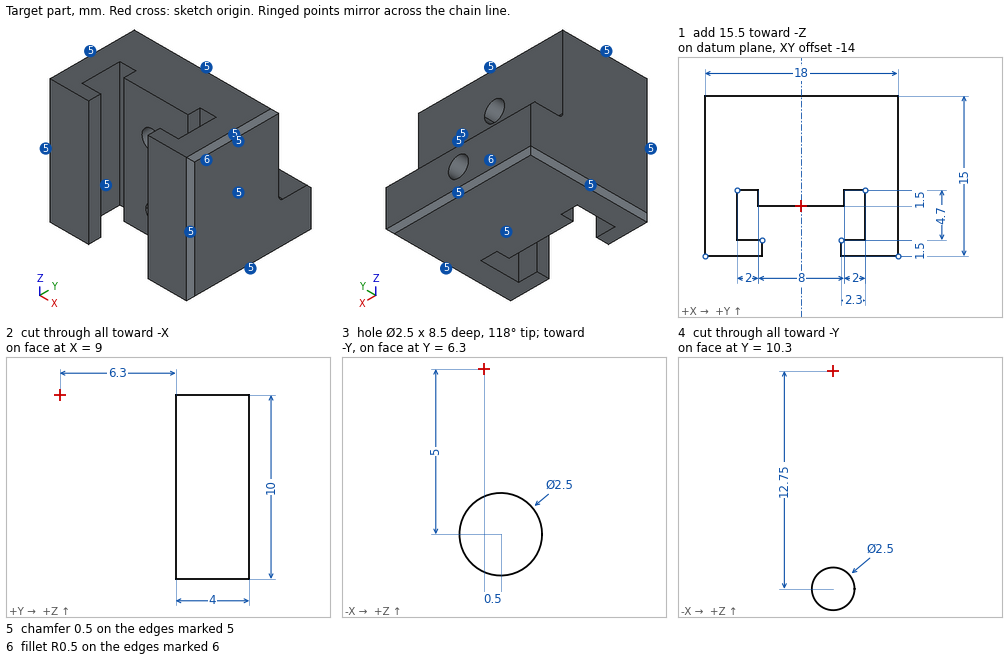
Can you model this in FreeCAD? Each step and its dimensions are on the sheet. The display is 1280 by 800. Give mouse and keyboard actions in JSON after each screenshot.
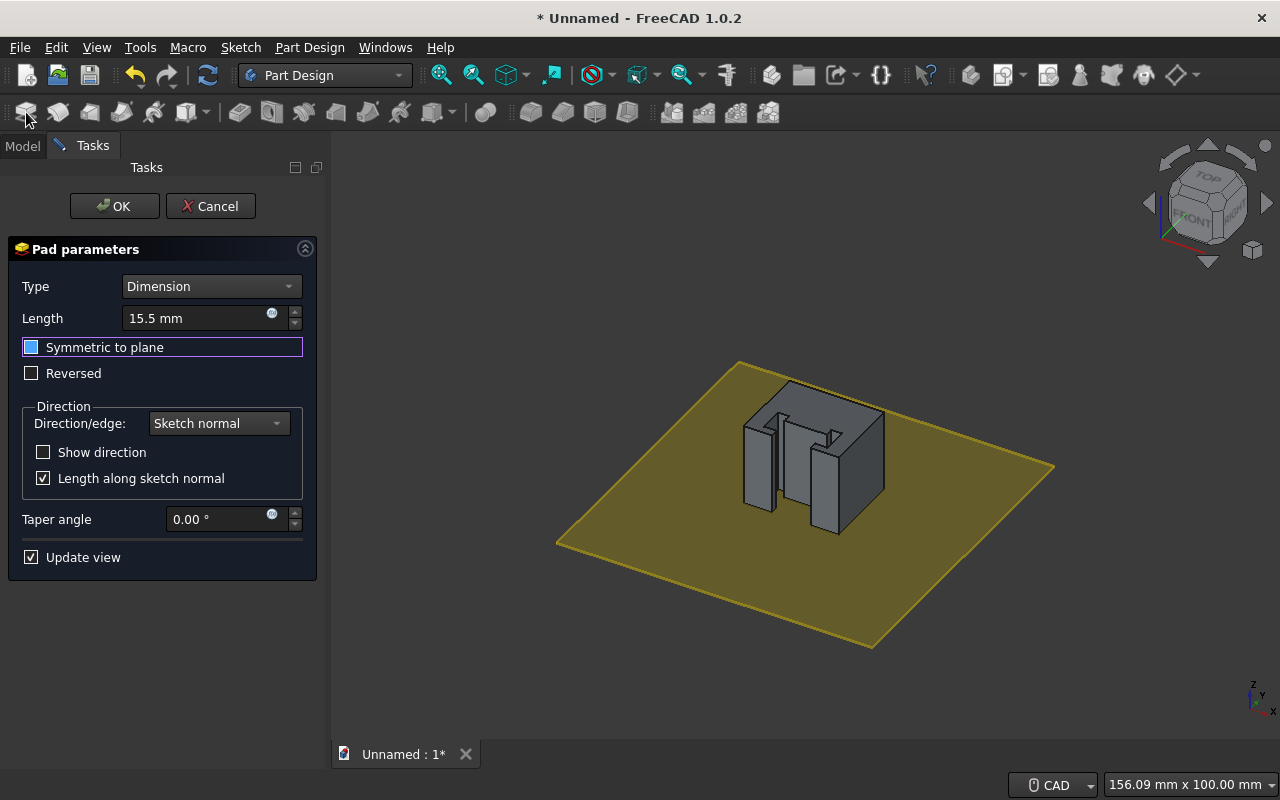
{"action": "left_click", "coordinate": [30, 373]}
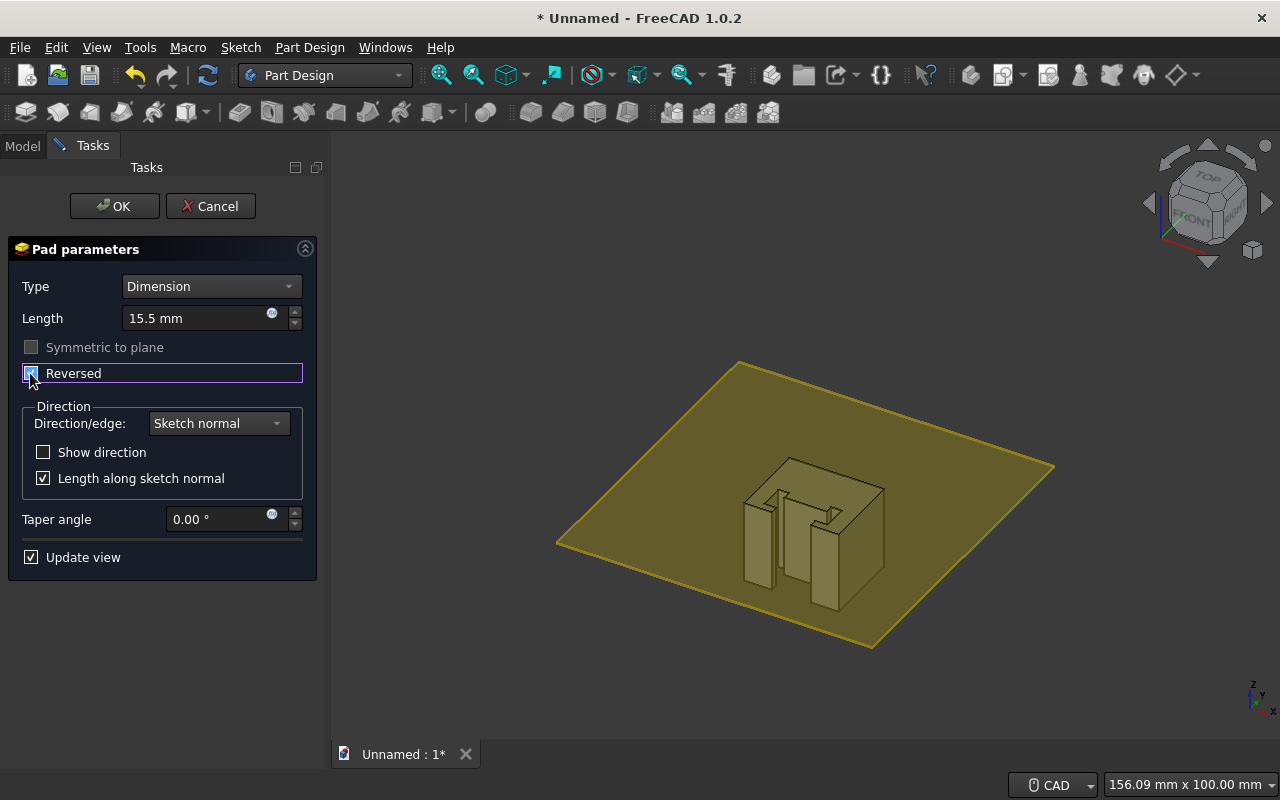
{"action": "left_click", "coordinate": [115, 206]}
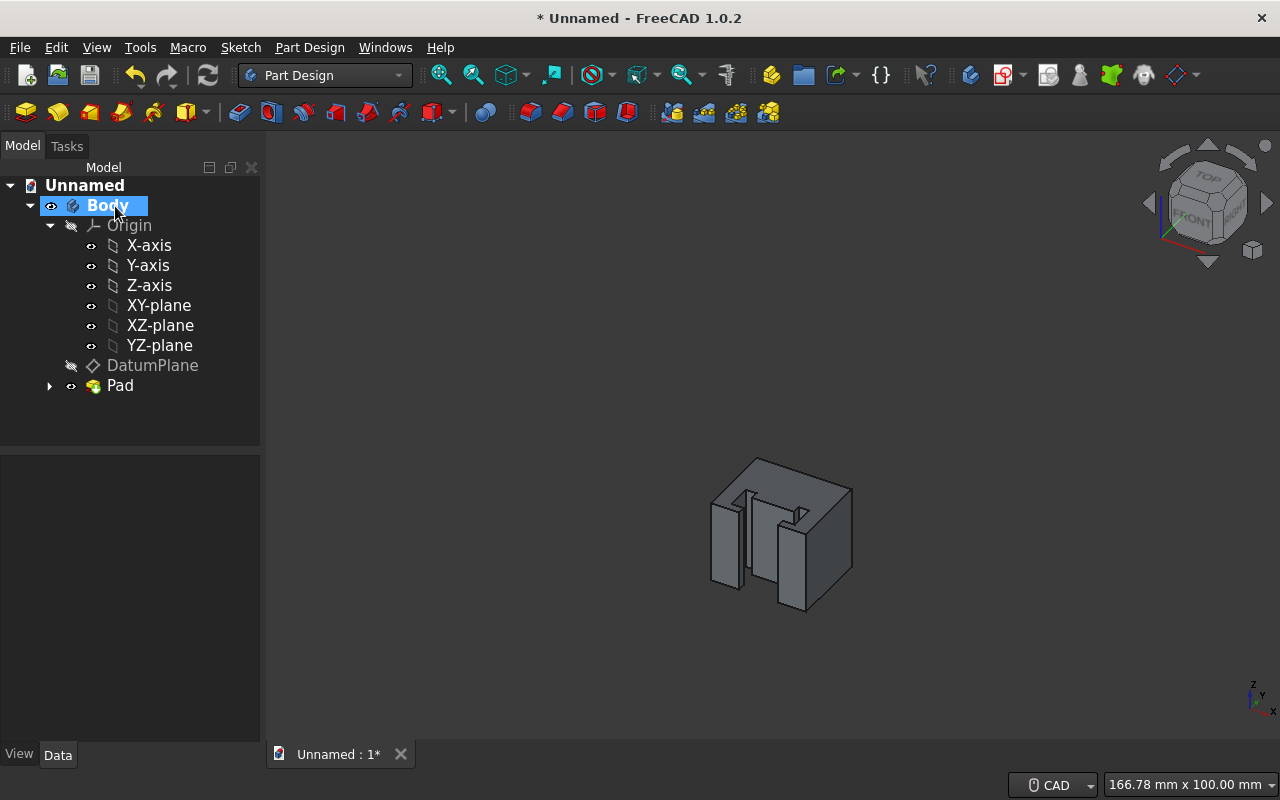
{"action": "left_click", "coordinate": [442, 76]}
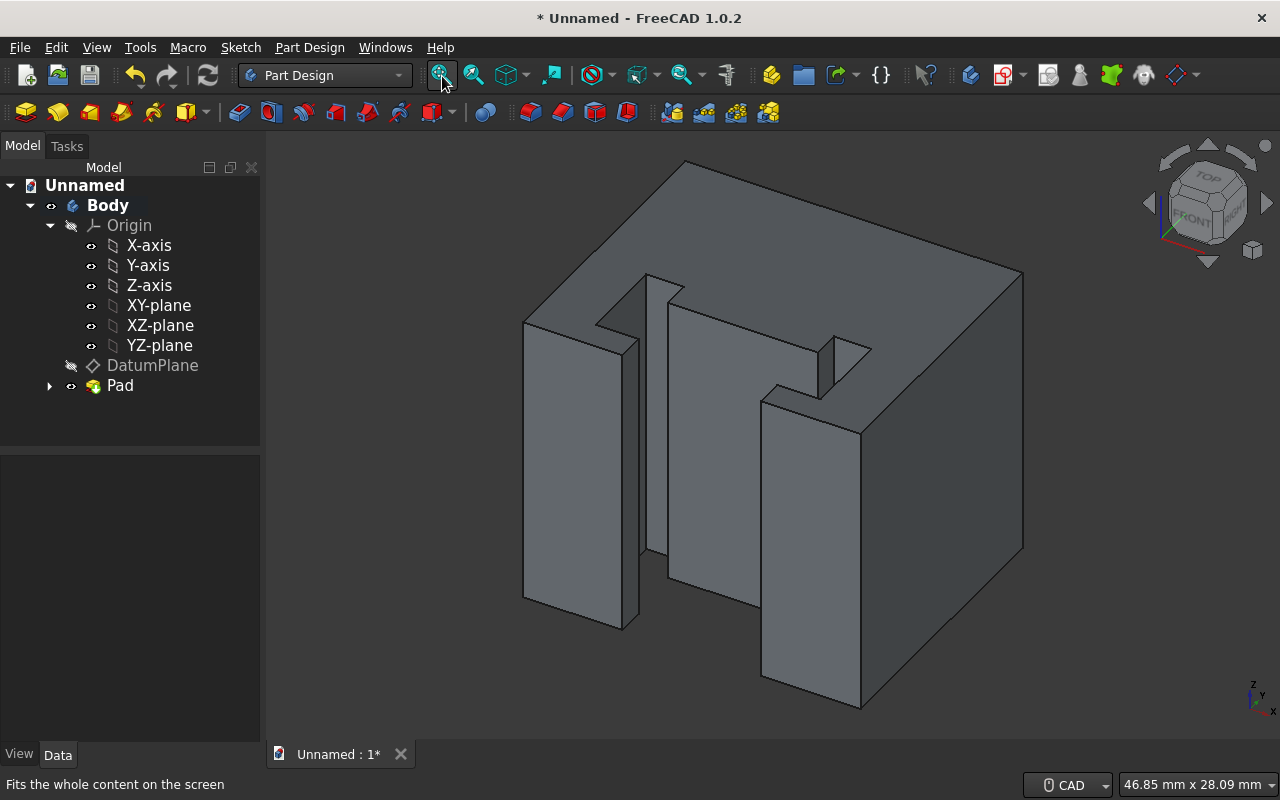
{"action": "left_click", "coordinate": [942, 490]}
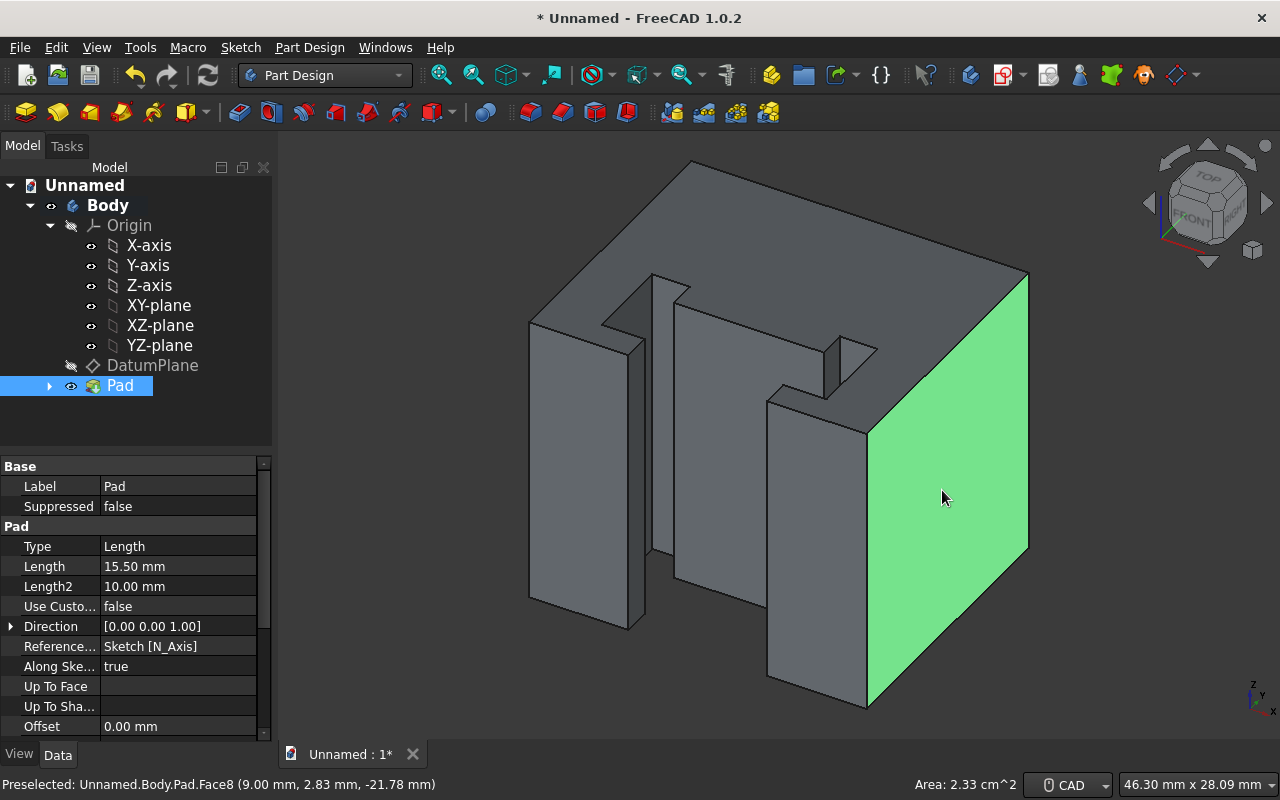
{"action": "left_click", "coordinate": [1004, 76]}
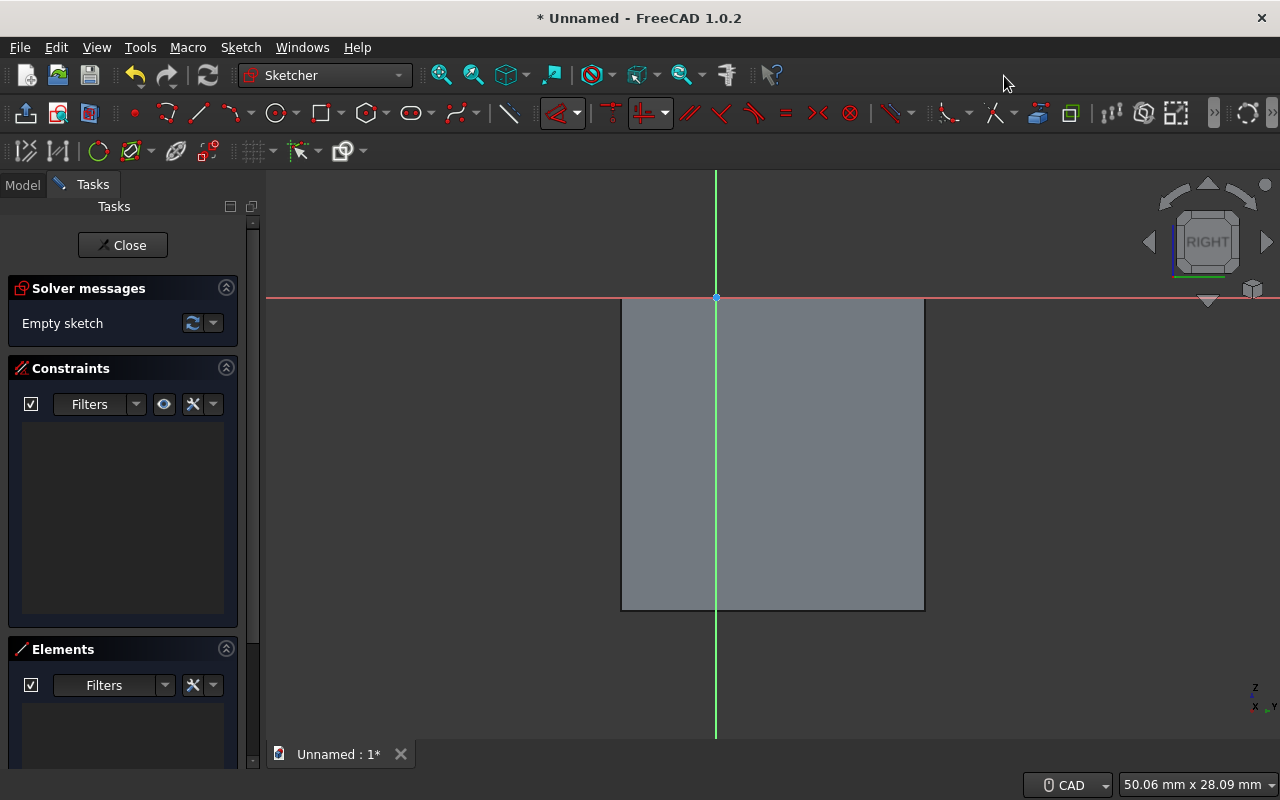
{"action": "scroll", "coordinate": [962, 331], "scroll_direction": "up", "scroll_amount": 3}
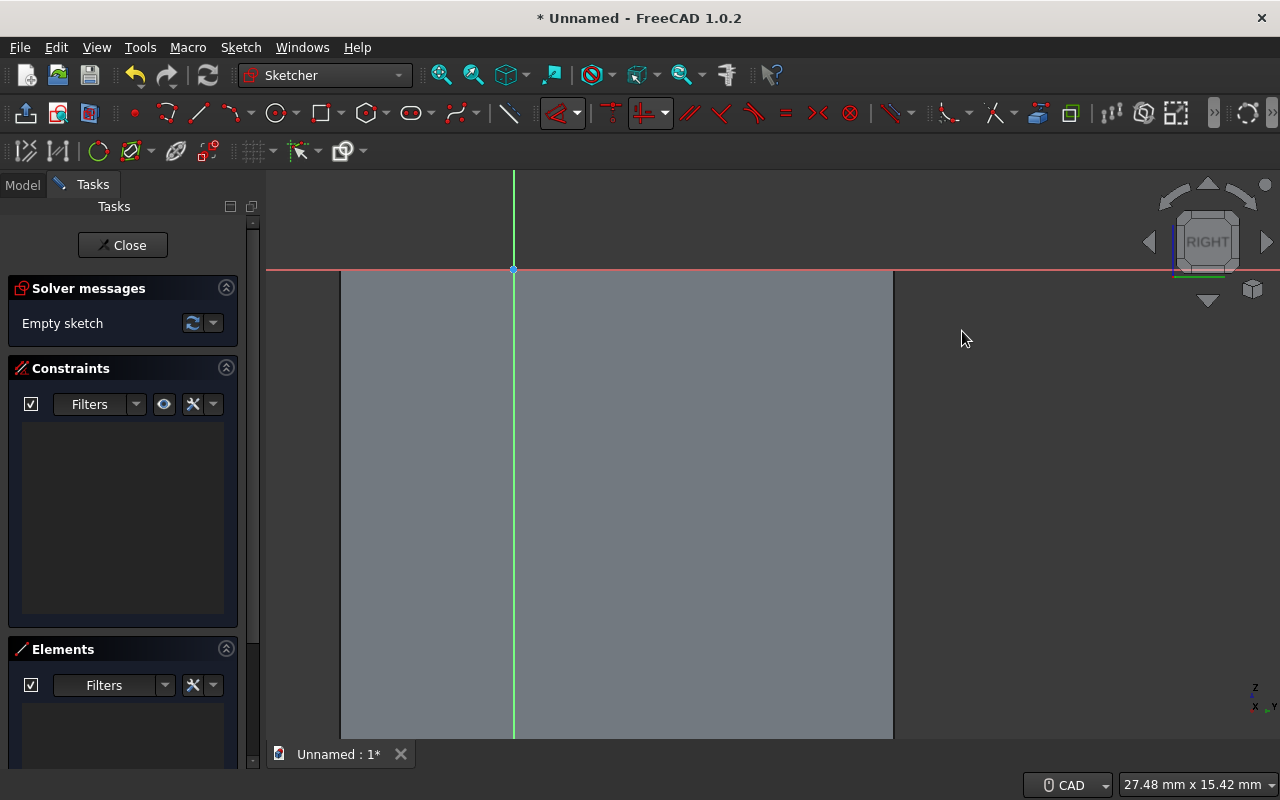
{"action": "key", "text": "g r"}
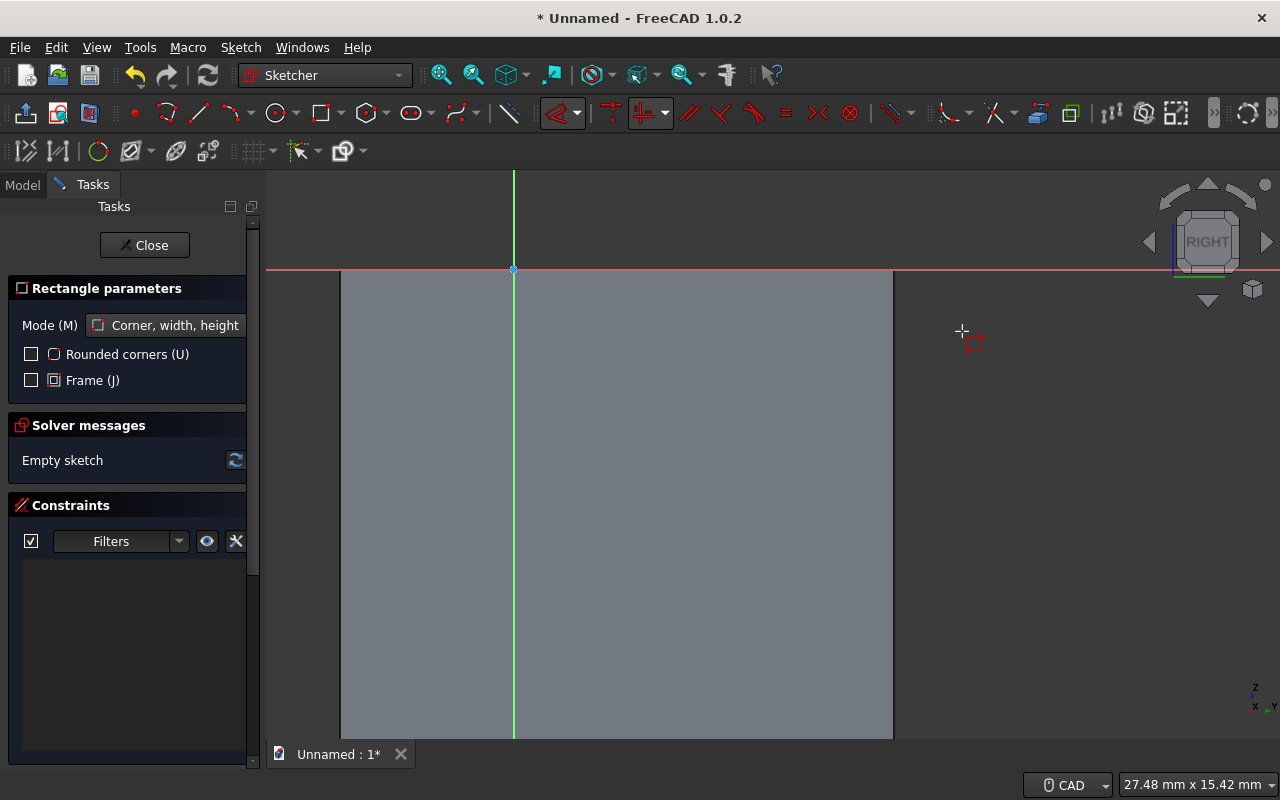
{"action": "left_click", "coordinate": [746, 270]}
{"action": "mouse_move", "coordinate": [894, 639]}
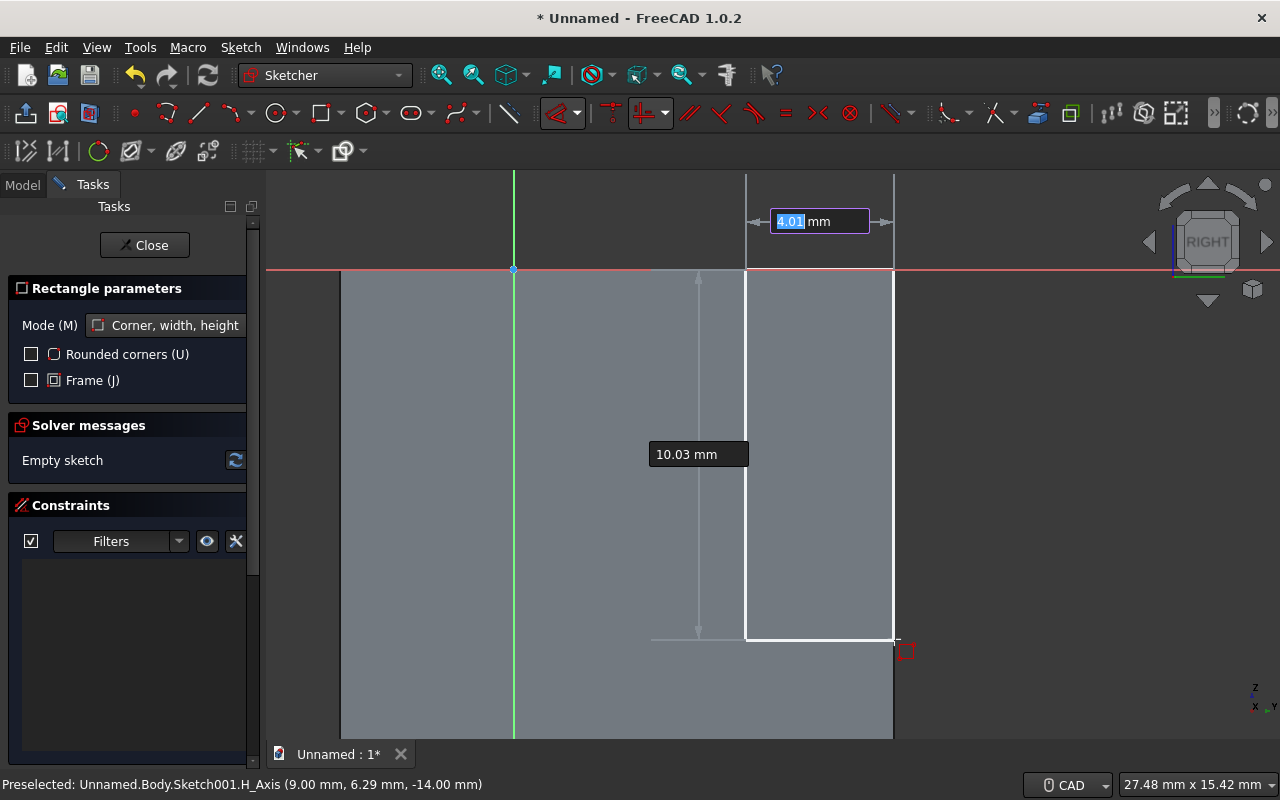
{"action": "type", "text": "4"}
{"action": "key", "text": "Tab"}
{"action": "type", "text": "10"}
{"action": "key", "text": "Return"}
{"action": "key", "text": "Escape"}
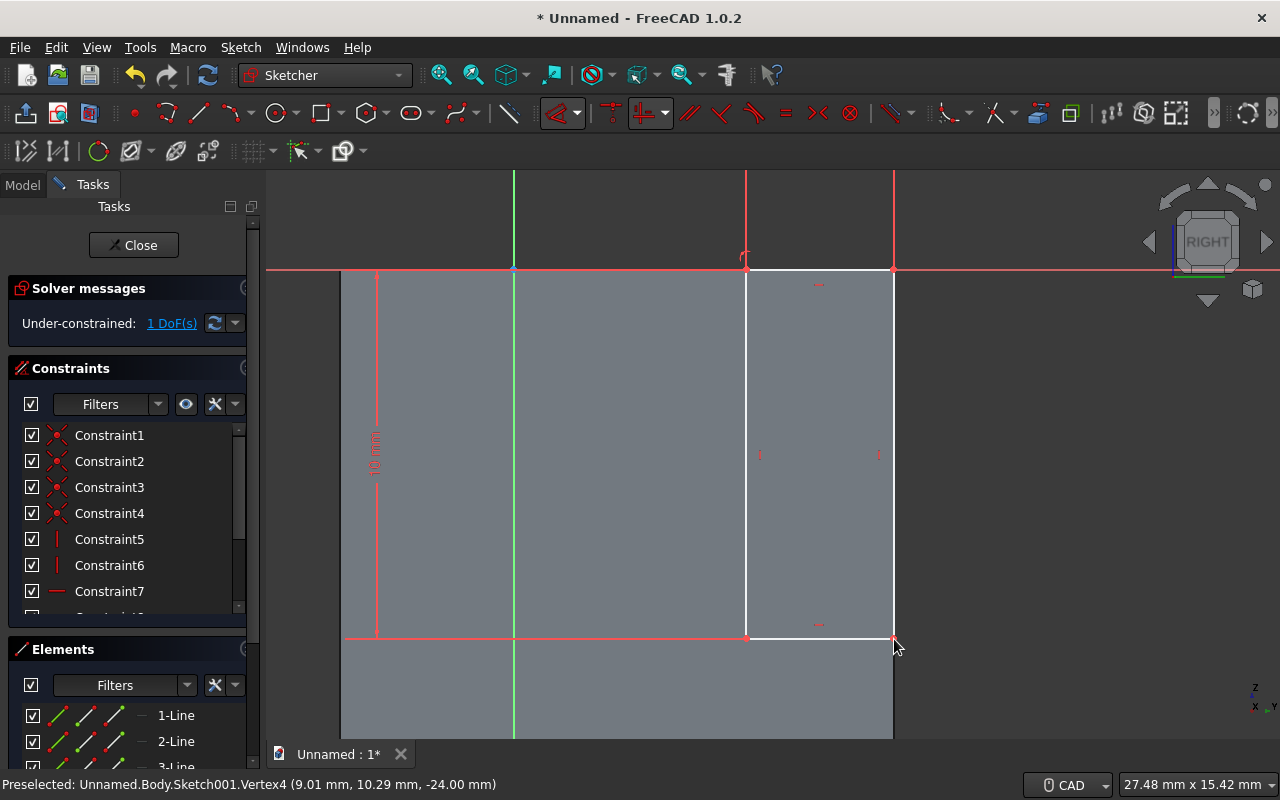
{"action": "key", "text": "d"}